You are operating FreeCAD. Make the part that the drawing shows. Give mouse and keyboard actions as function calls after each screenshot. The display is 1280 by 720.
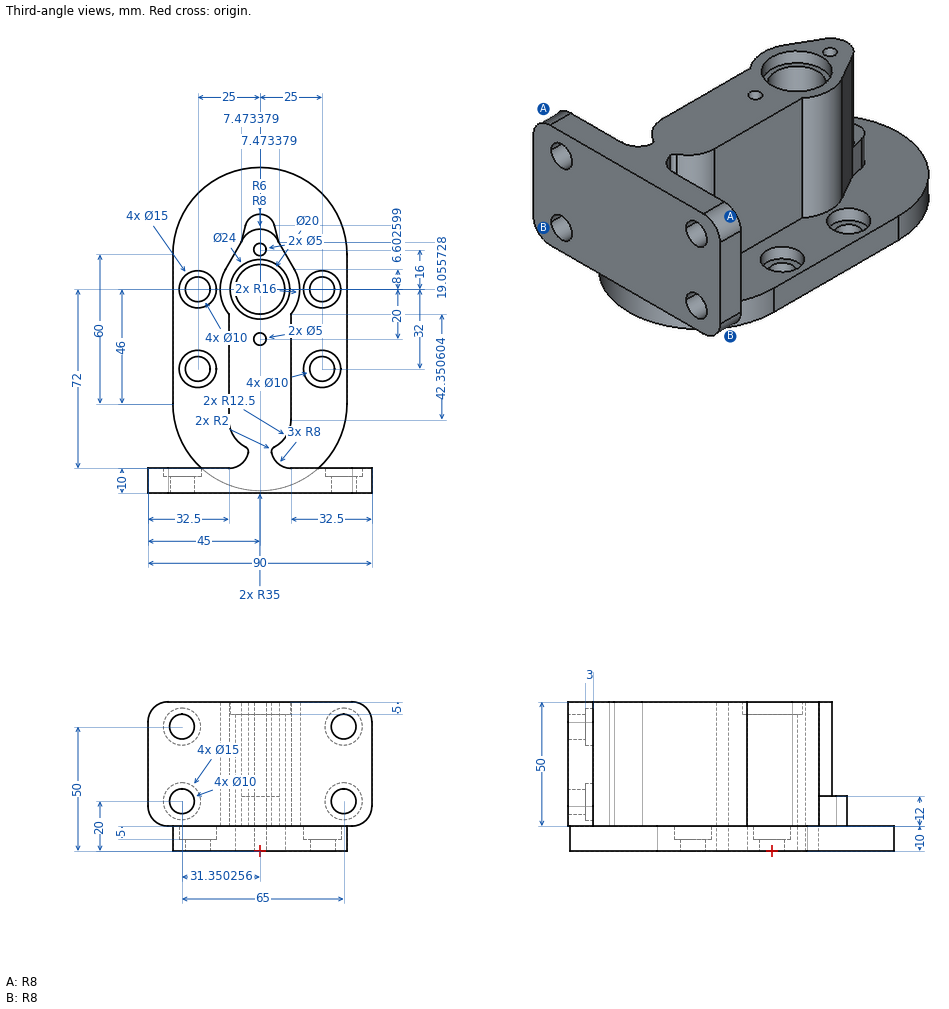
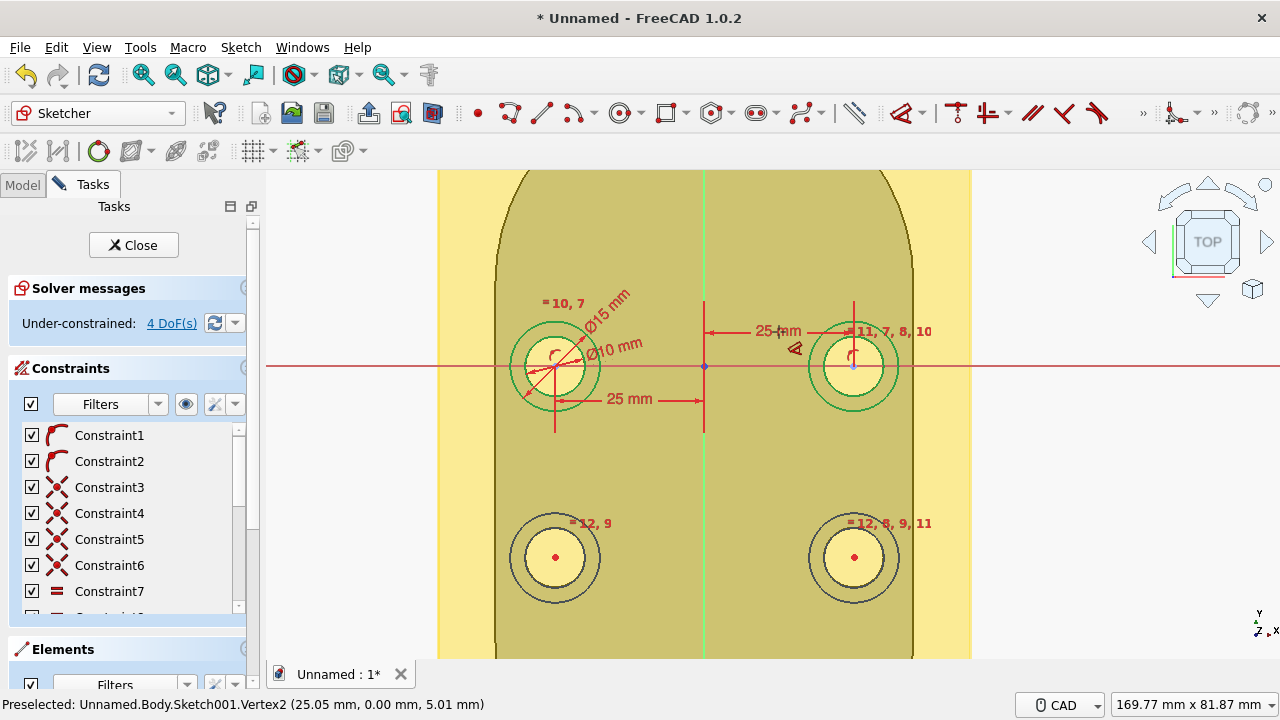
click(854, 558)
click(779, 592)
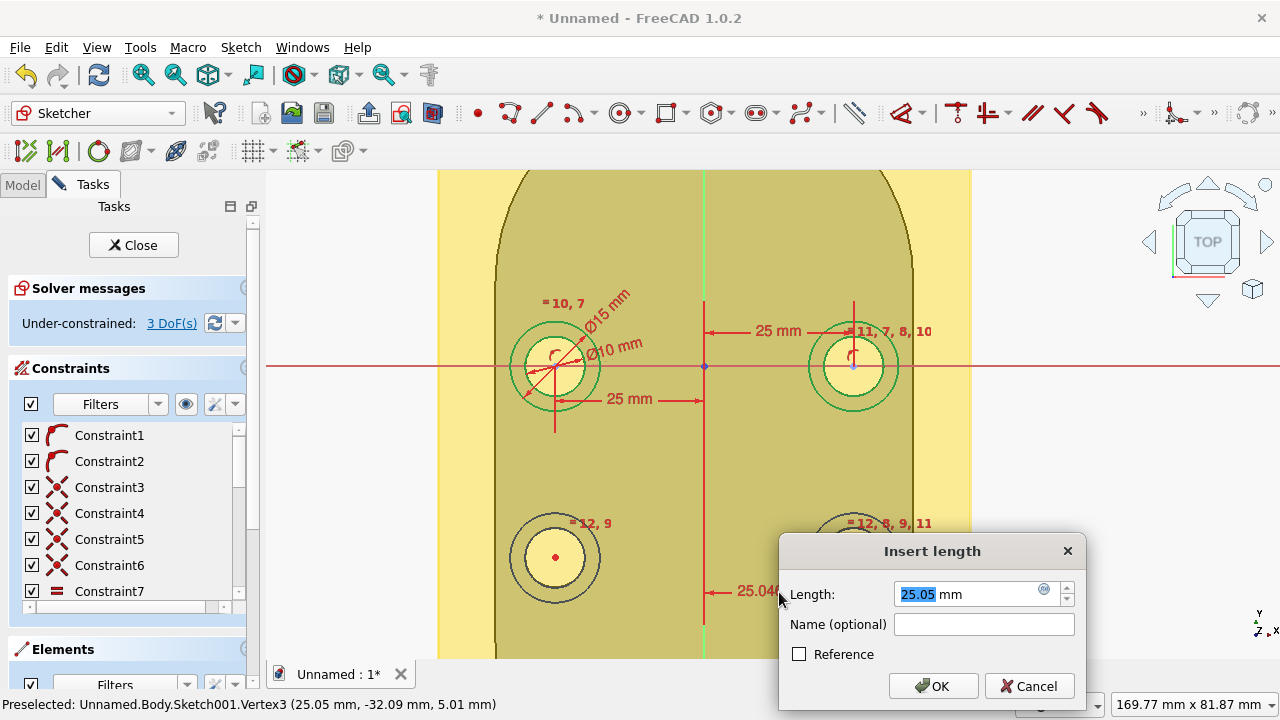
text(25)
key(Return)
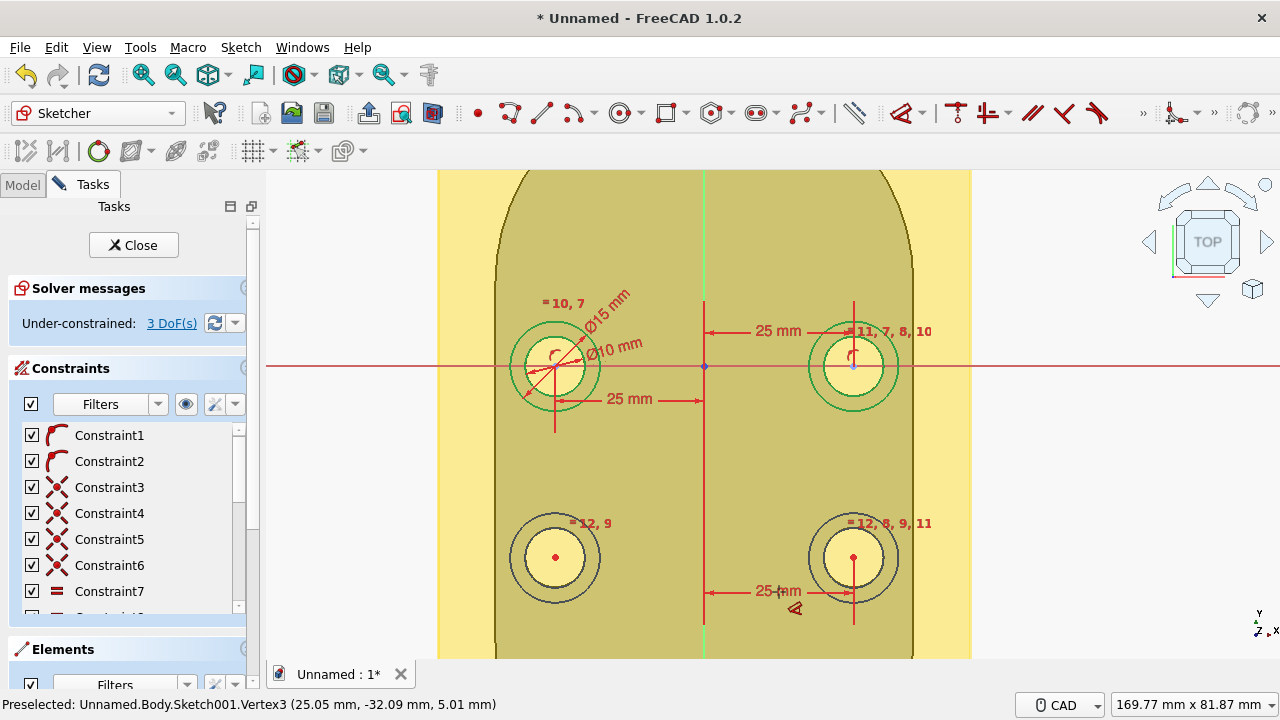
click(854, 558)
click(888, 462)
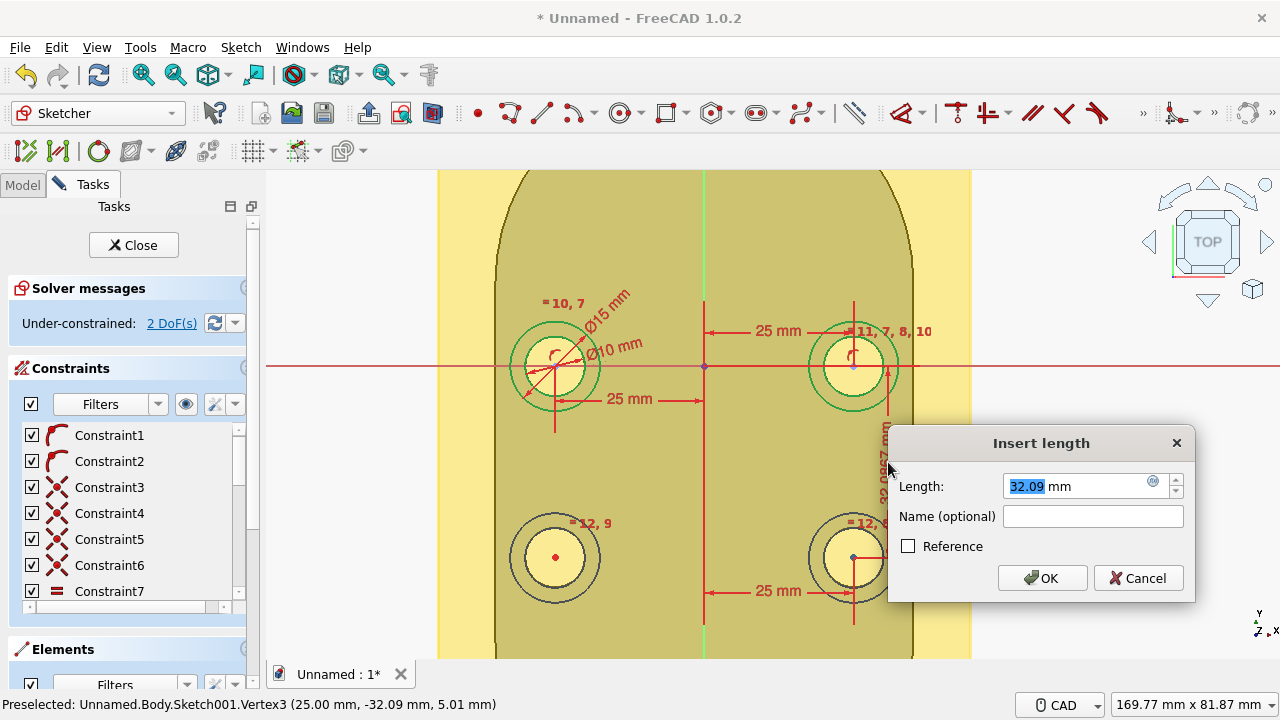
text(32)
key(Return)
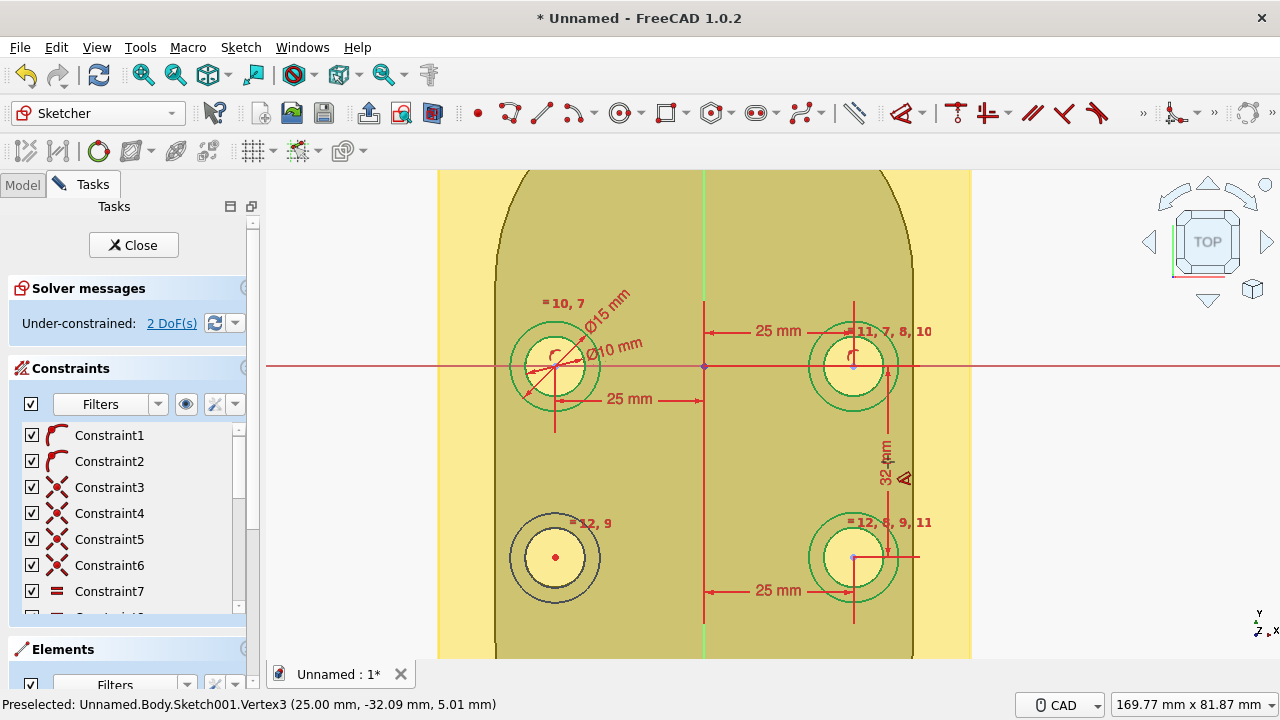
click(555, 558)
click(630, 592)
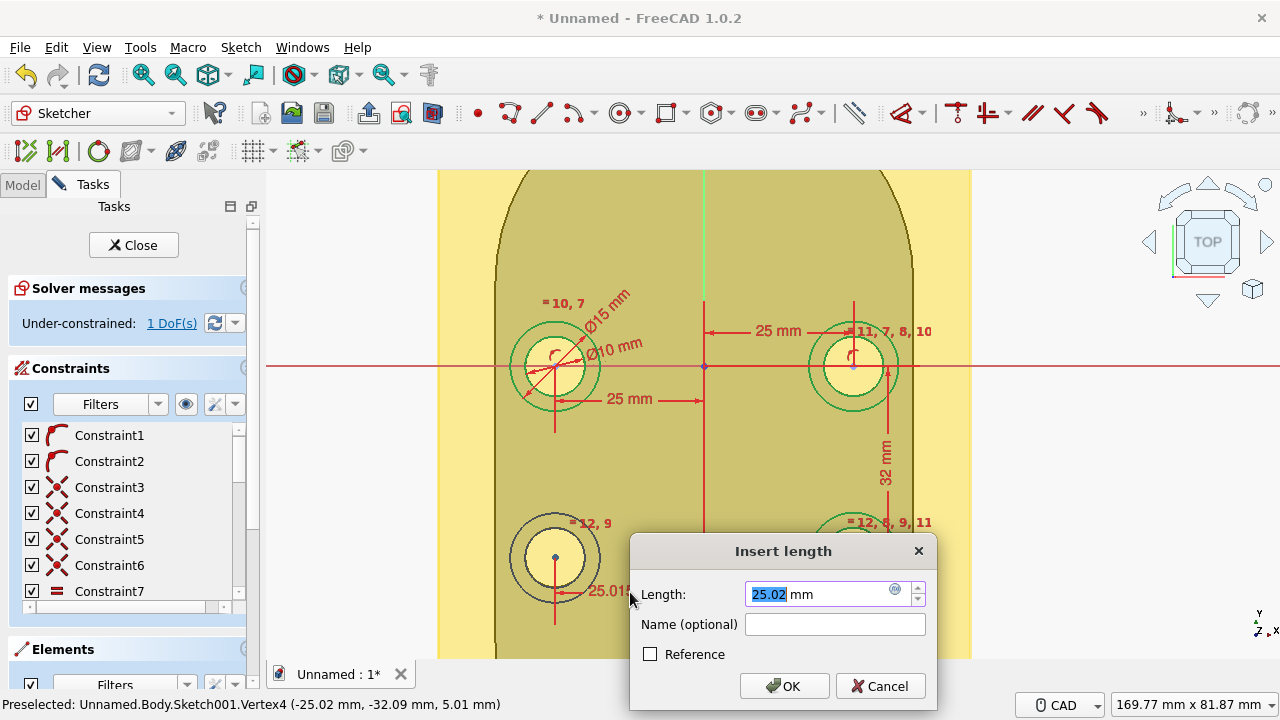
text(25)
key(Return)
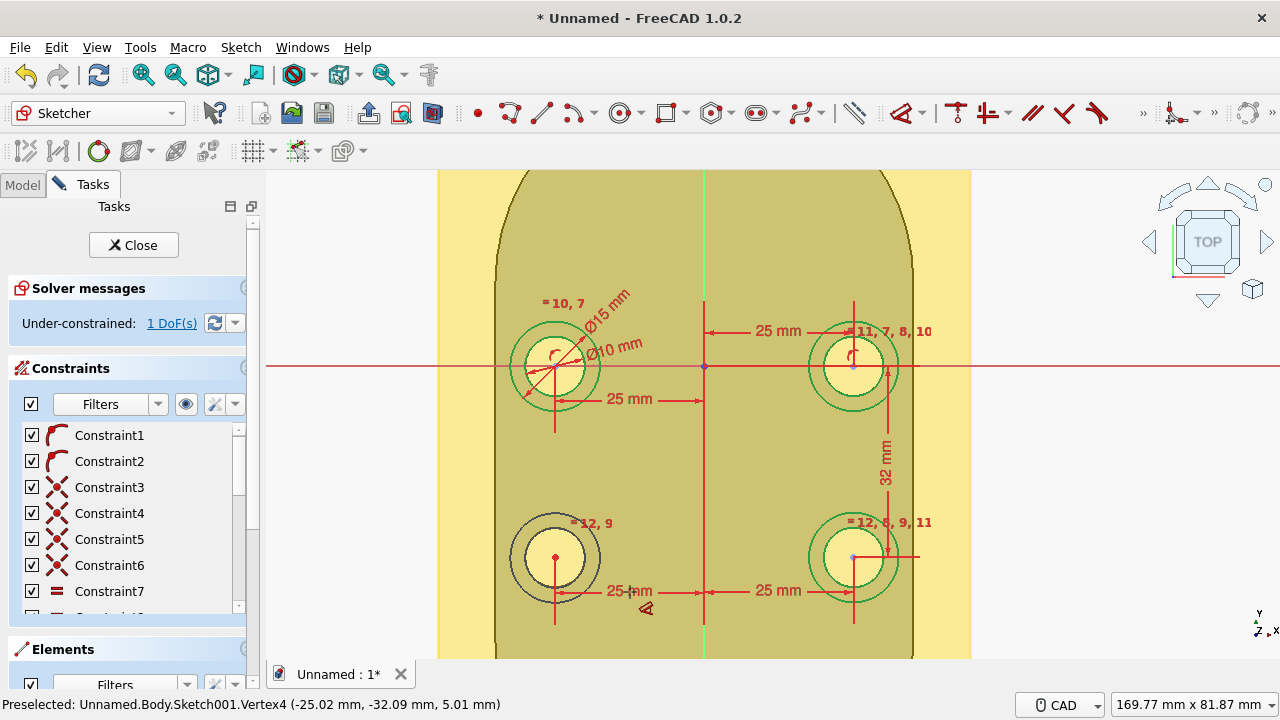
click(555, 558)
click(521, 462)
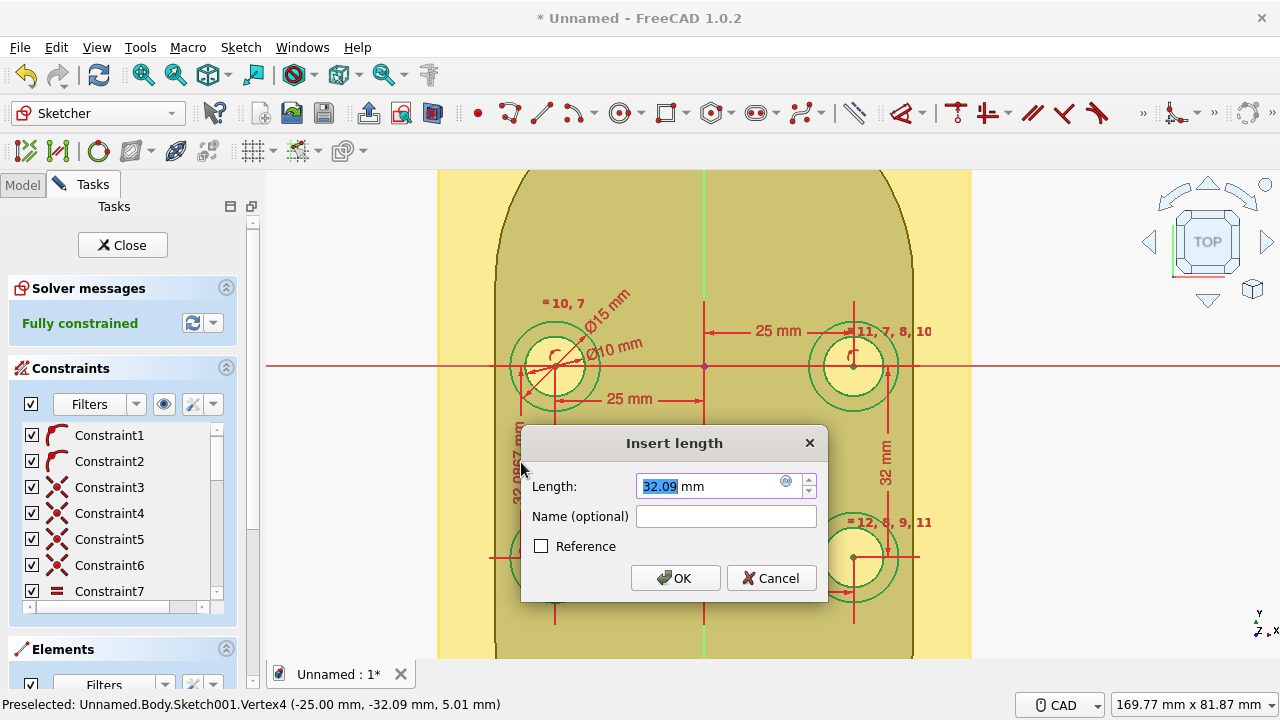
text(32)
key(Return)
key(Escape)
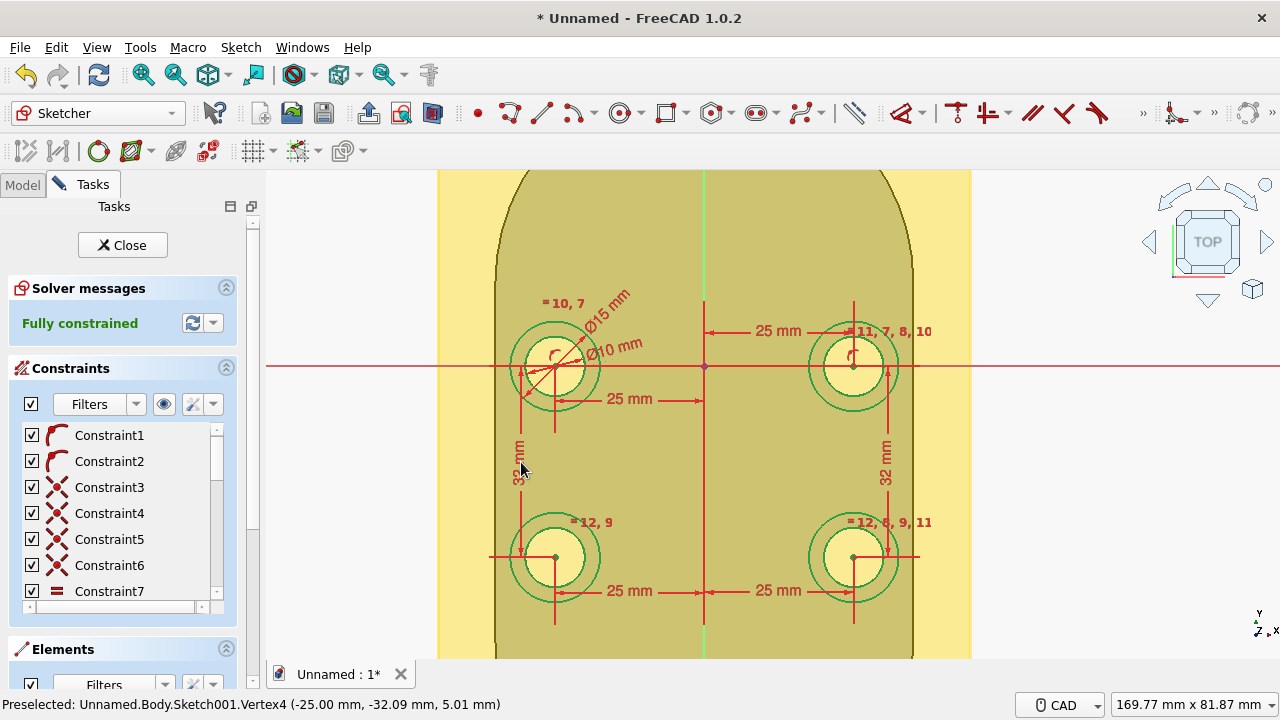
click(123, 245)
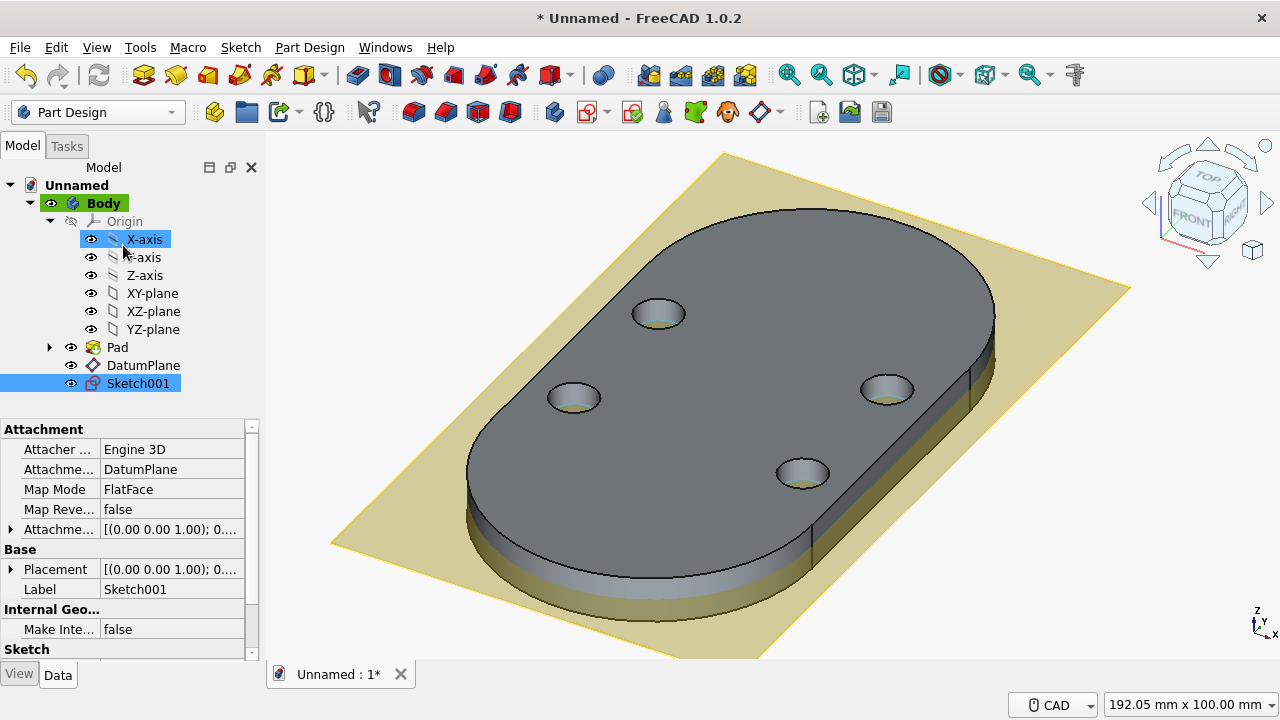
click(358, 76)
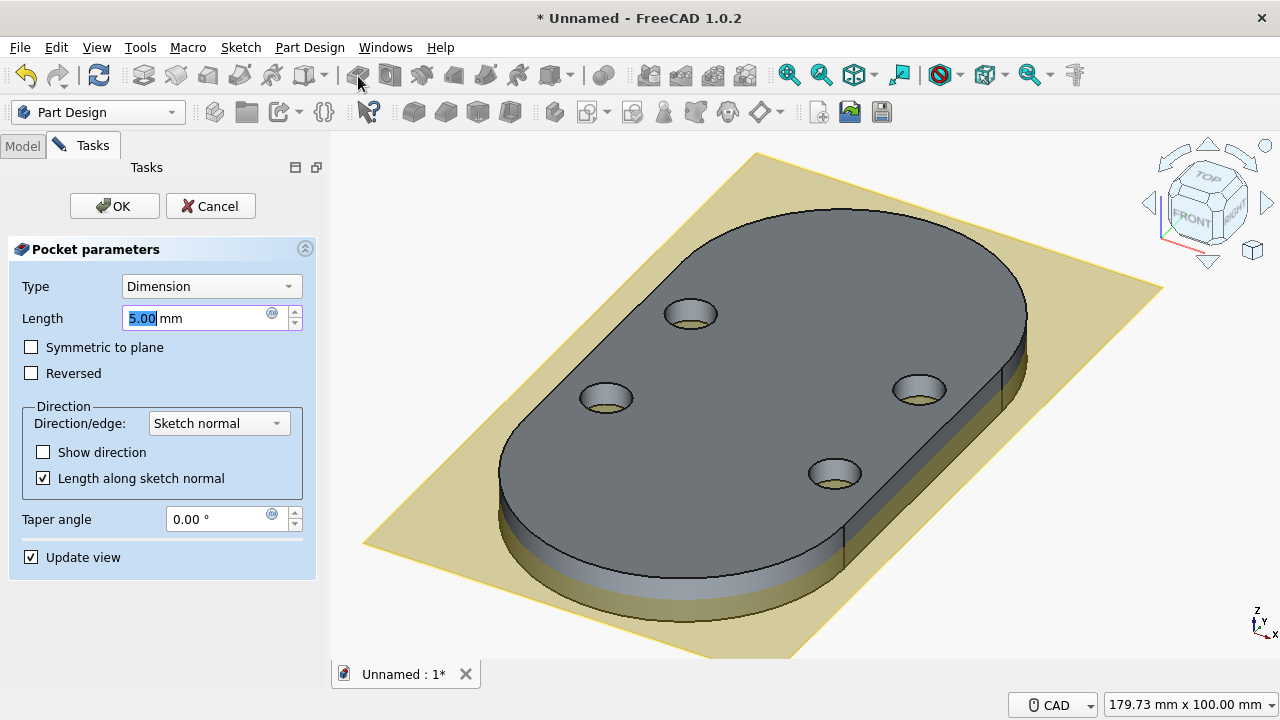
text(5)
key(Tab)